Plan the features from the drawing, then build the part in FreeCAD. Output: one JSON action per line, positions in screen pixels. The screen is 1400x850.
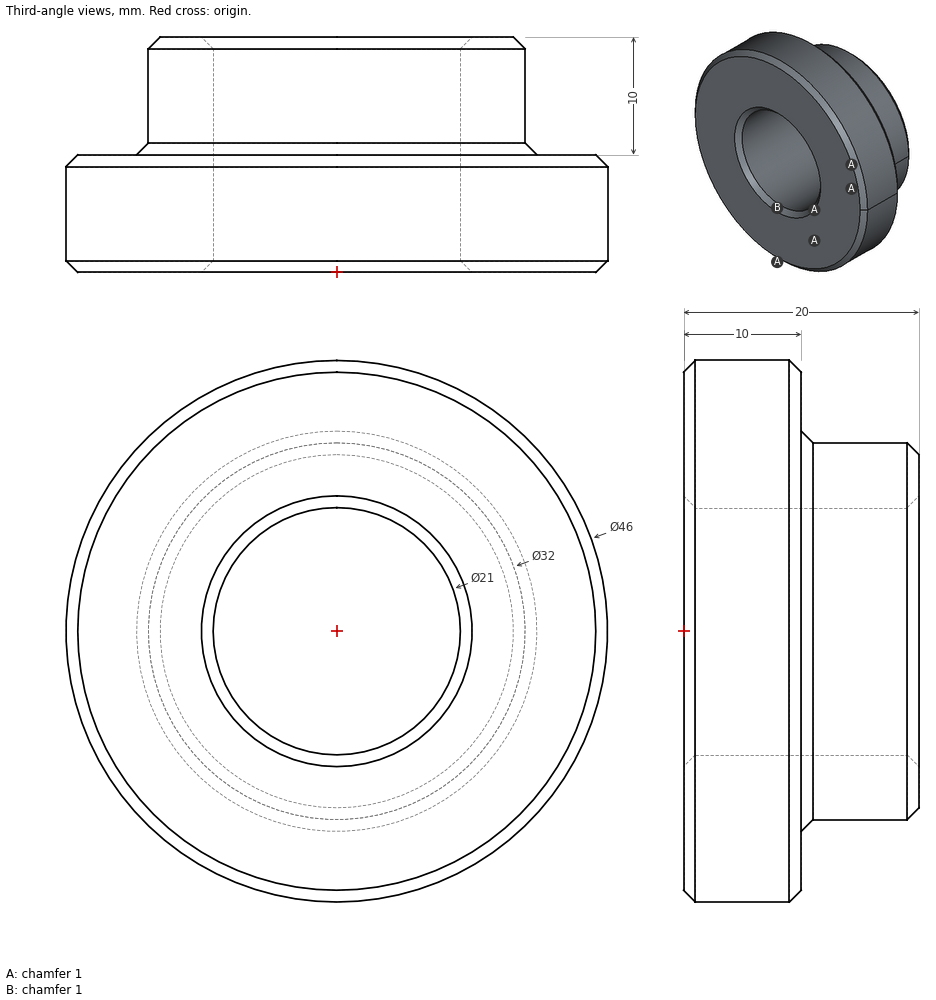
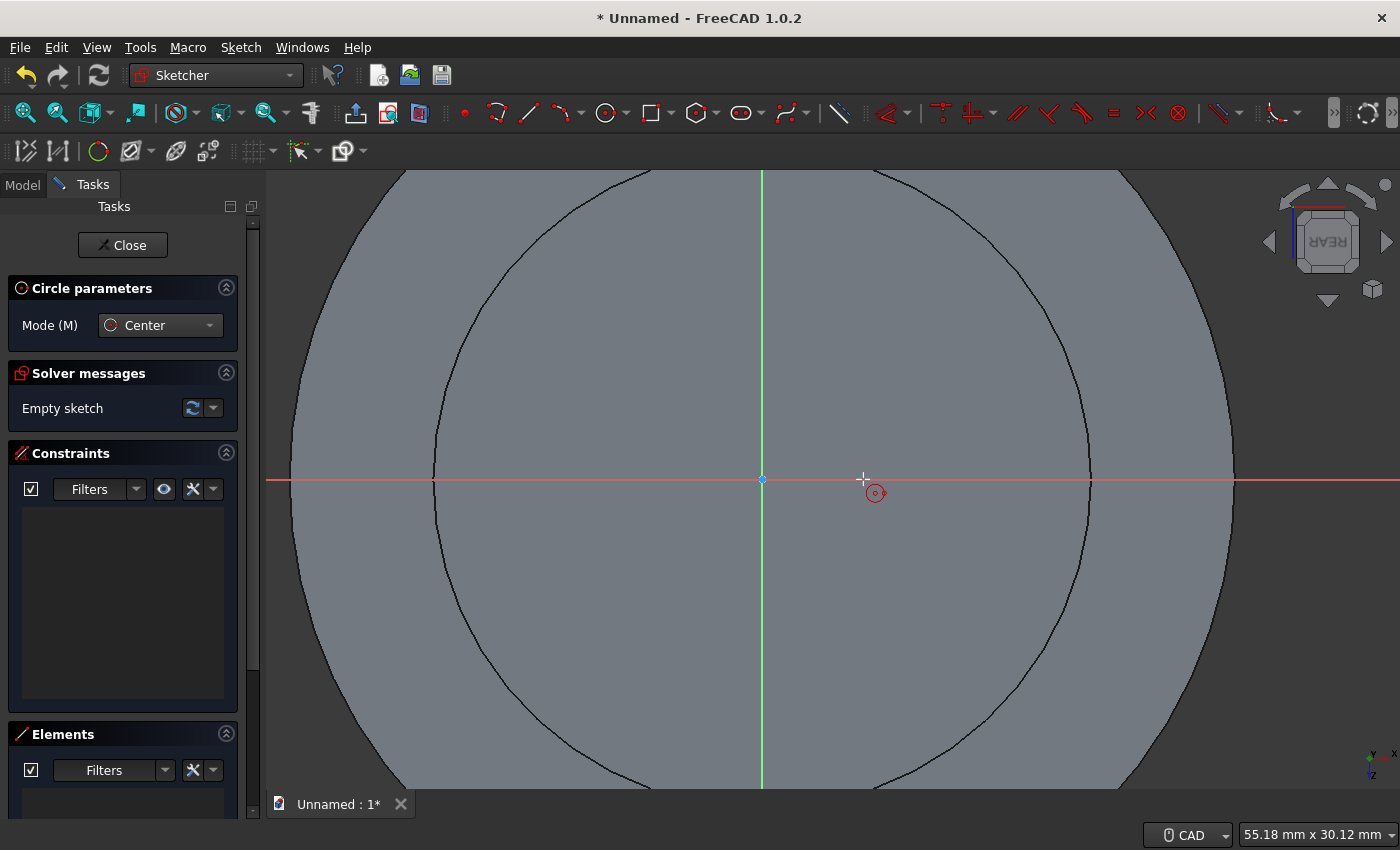
{"action": "left_click", "coordinate": [762, 479]}
{"action": "left_click", "coordinate": [915, 327]}
{"action": "key", "text": "Escape"}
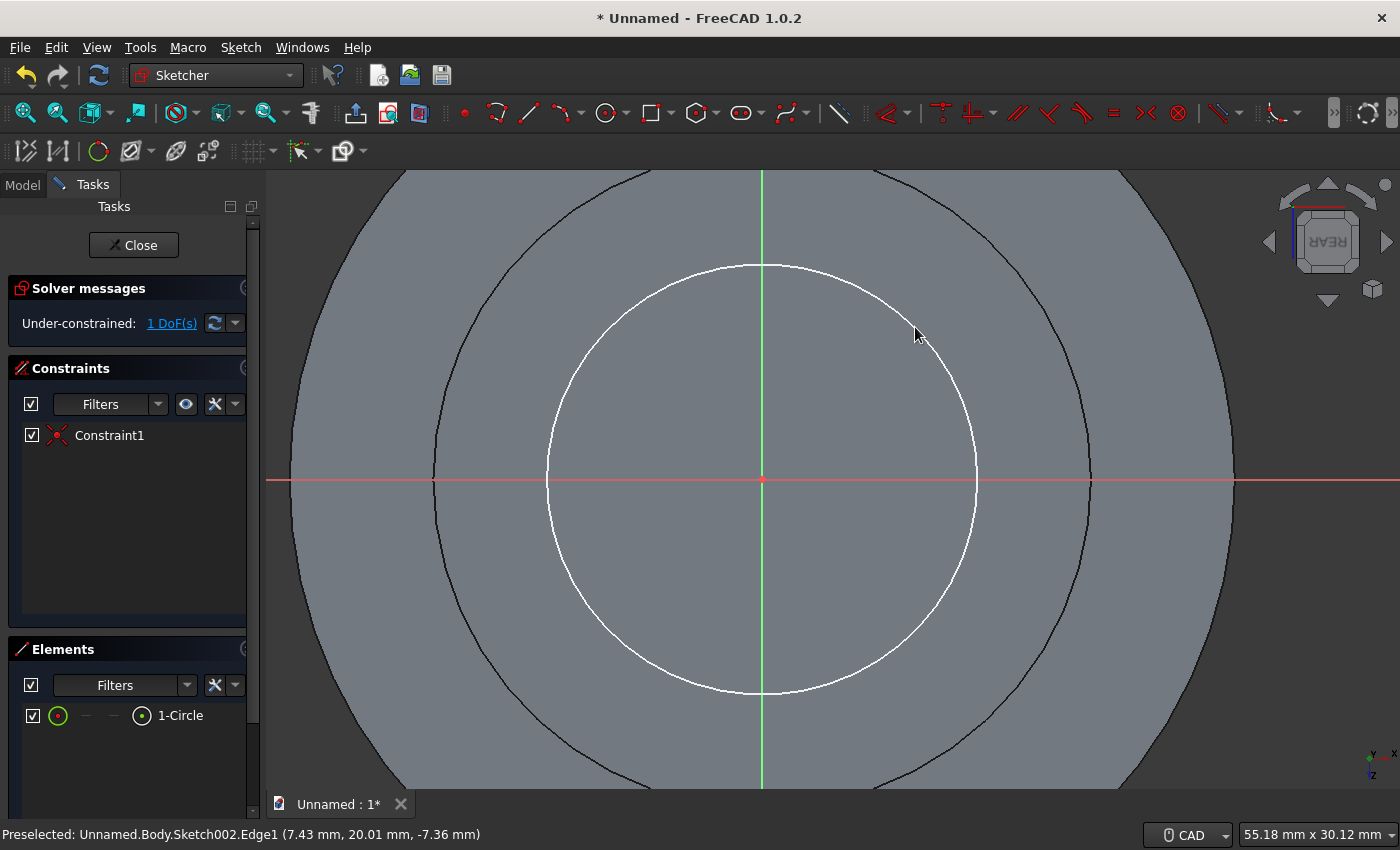
{"action": "key", "text": "d"}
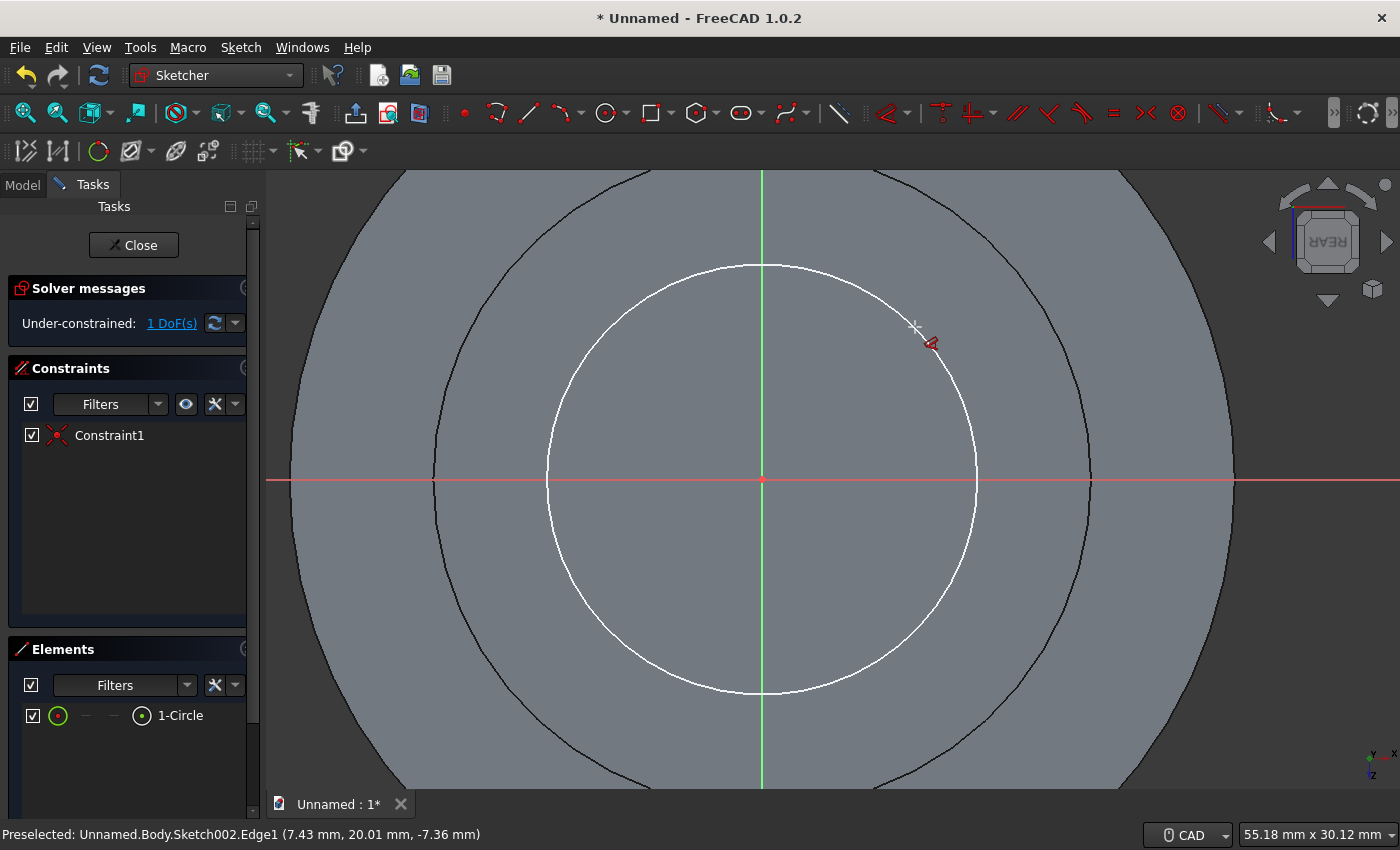
{"action": "left_click", "coordinate": [914, 327]}
{"action": "left_click", "coordinate": [937, 304]}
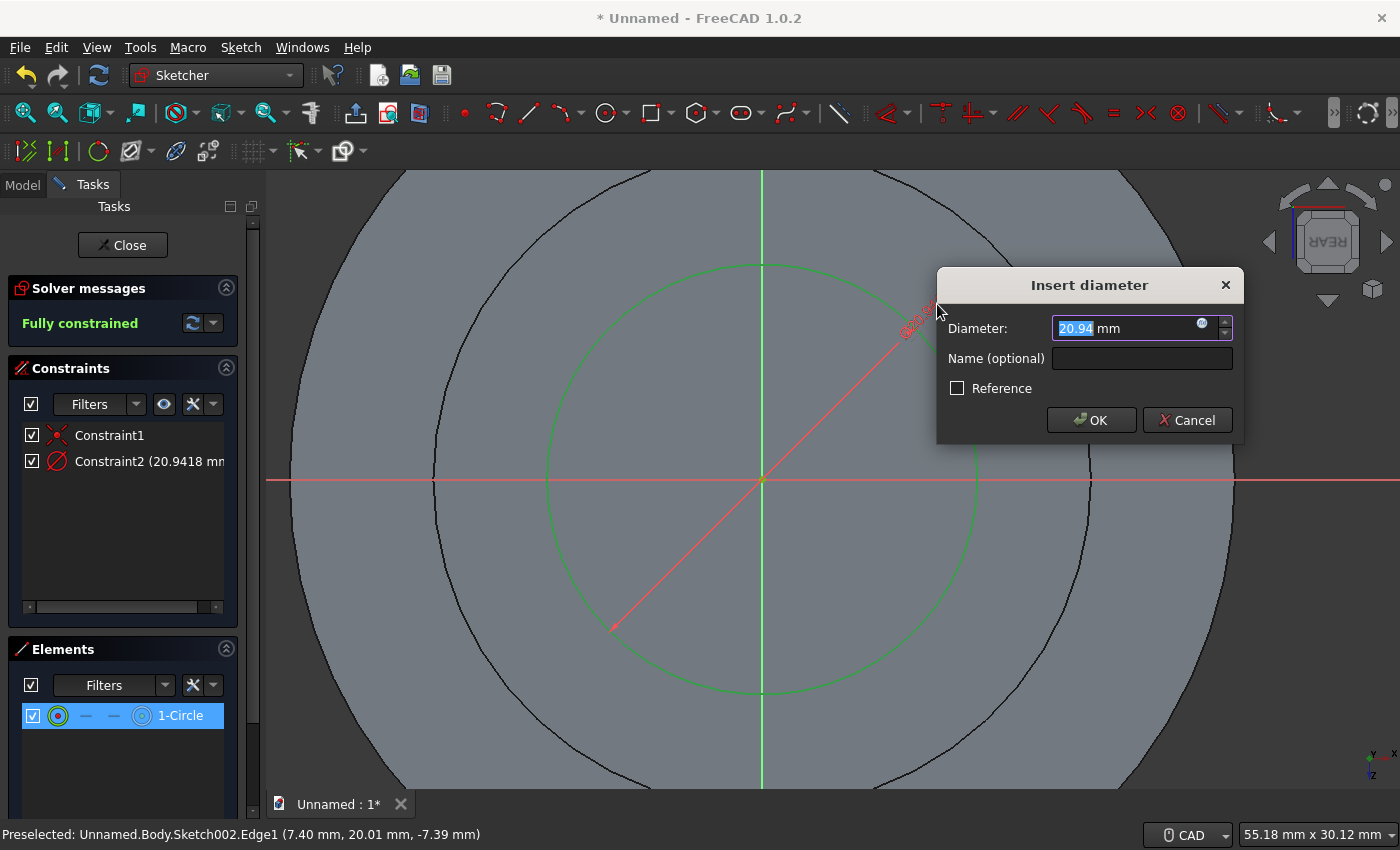
{"action": "type", "text": "21"}
{"action": "key", "text": "Return"}
{"action": "key", "text": "Escape"}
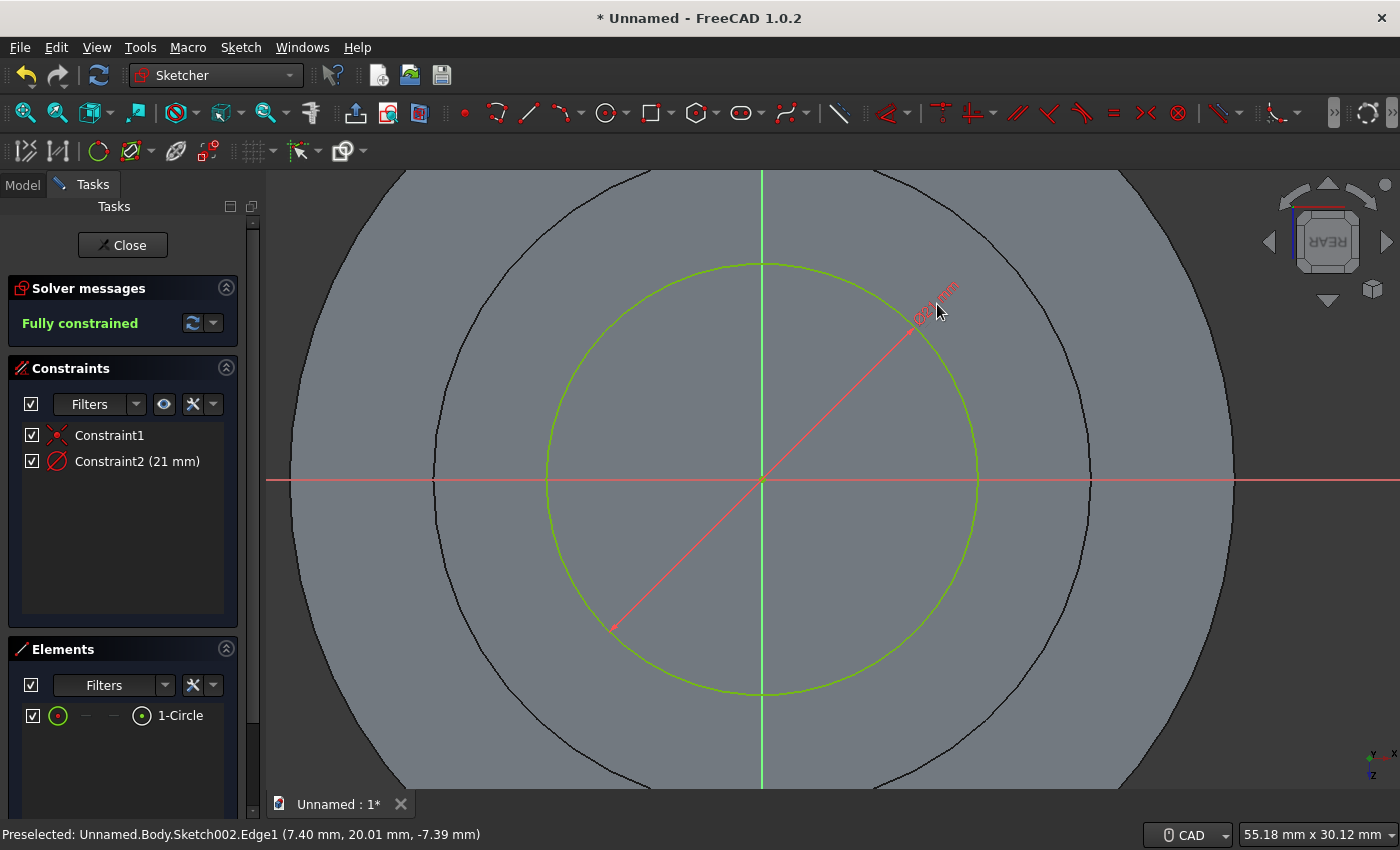
{"action": "left_click", "coordinate": [123, 245]}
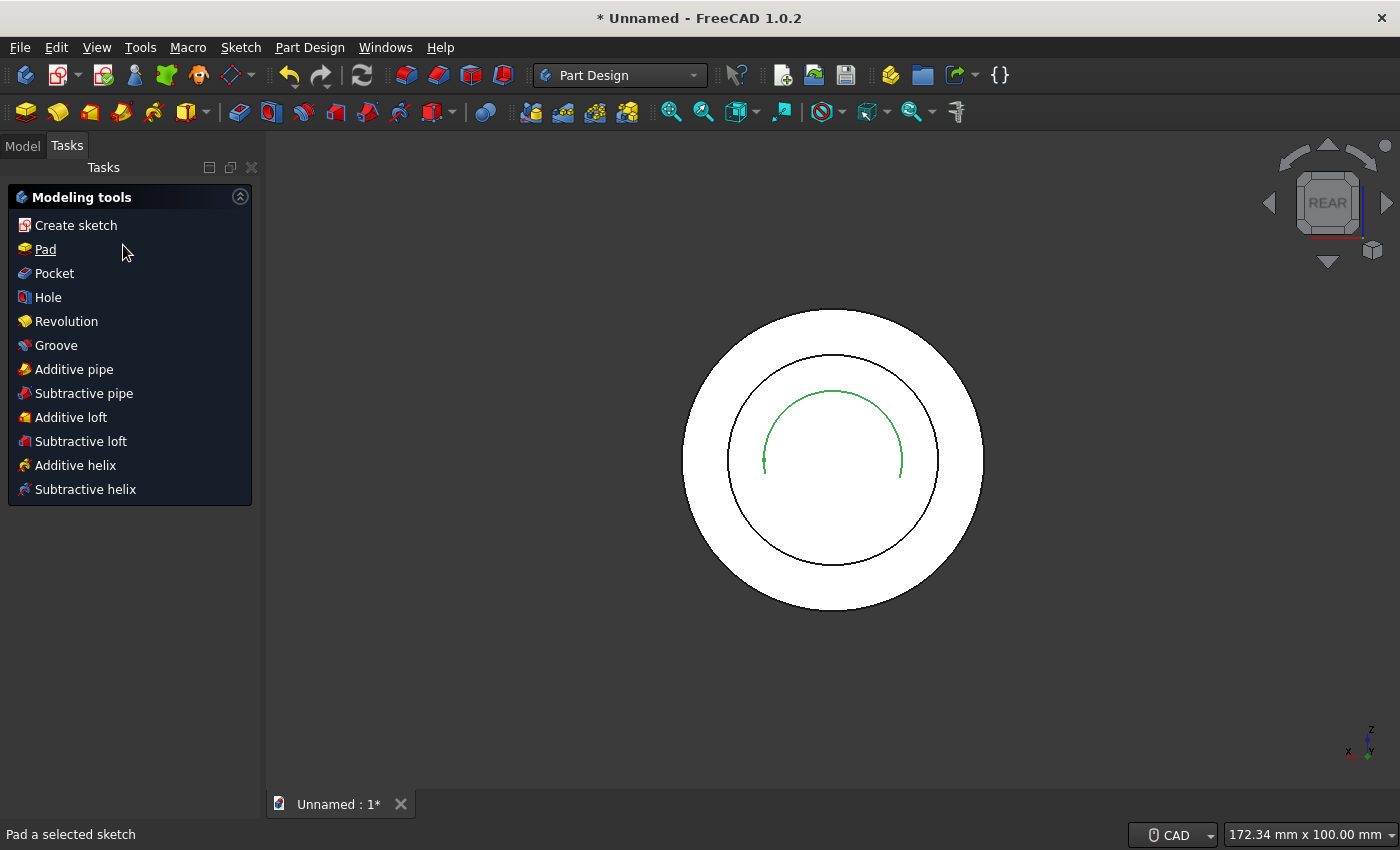
{"action": "left_click", "coordinate": [240, 112]}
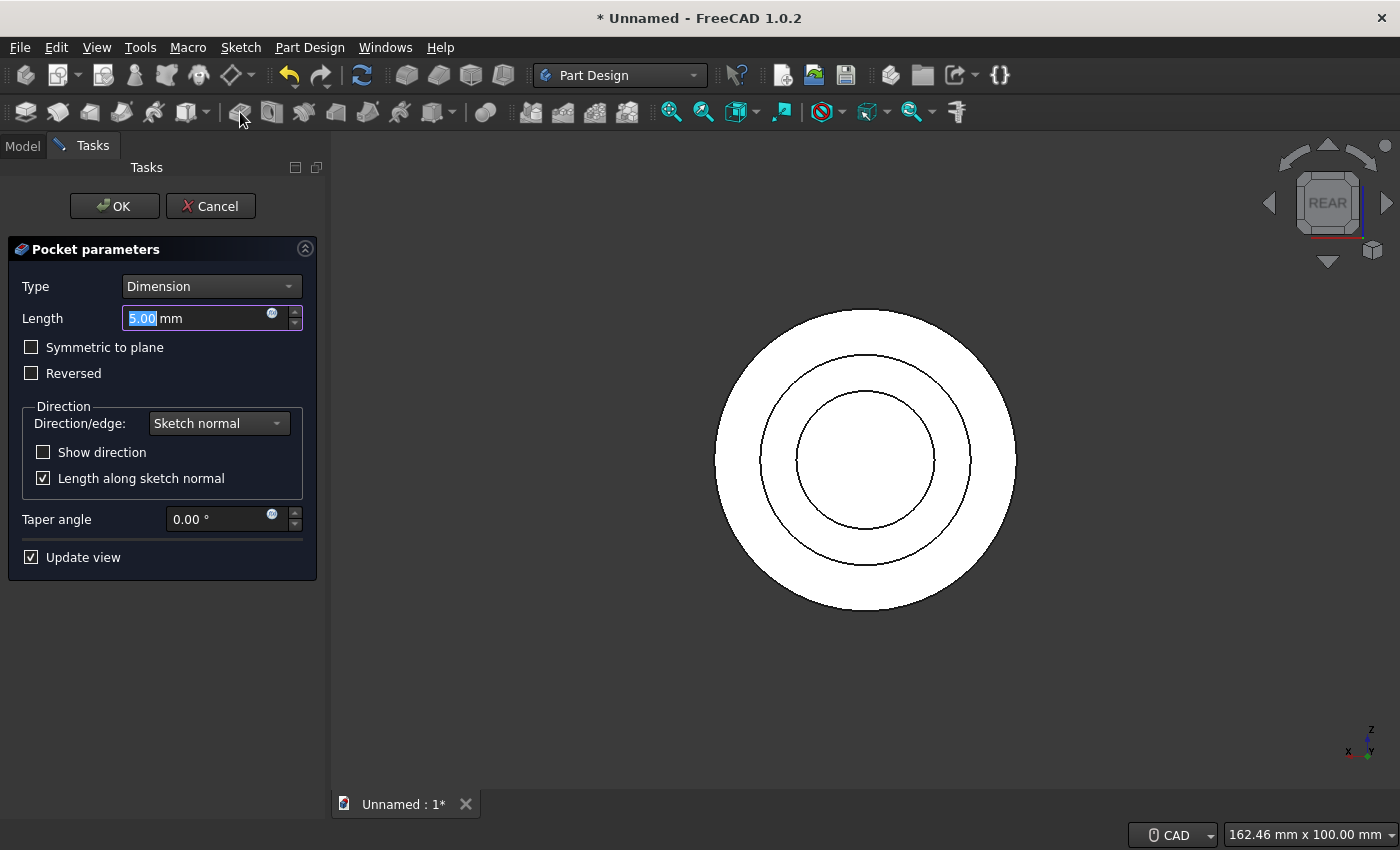
{"action": "type", "text": "20"}
{"action": "key", "text": "Tab"}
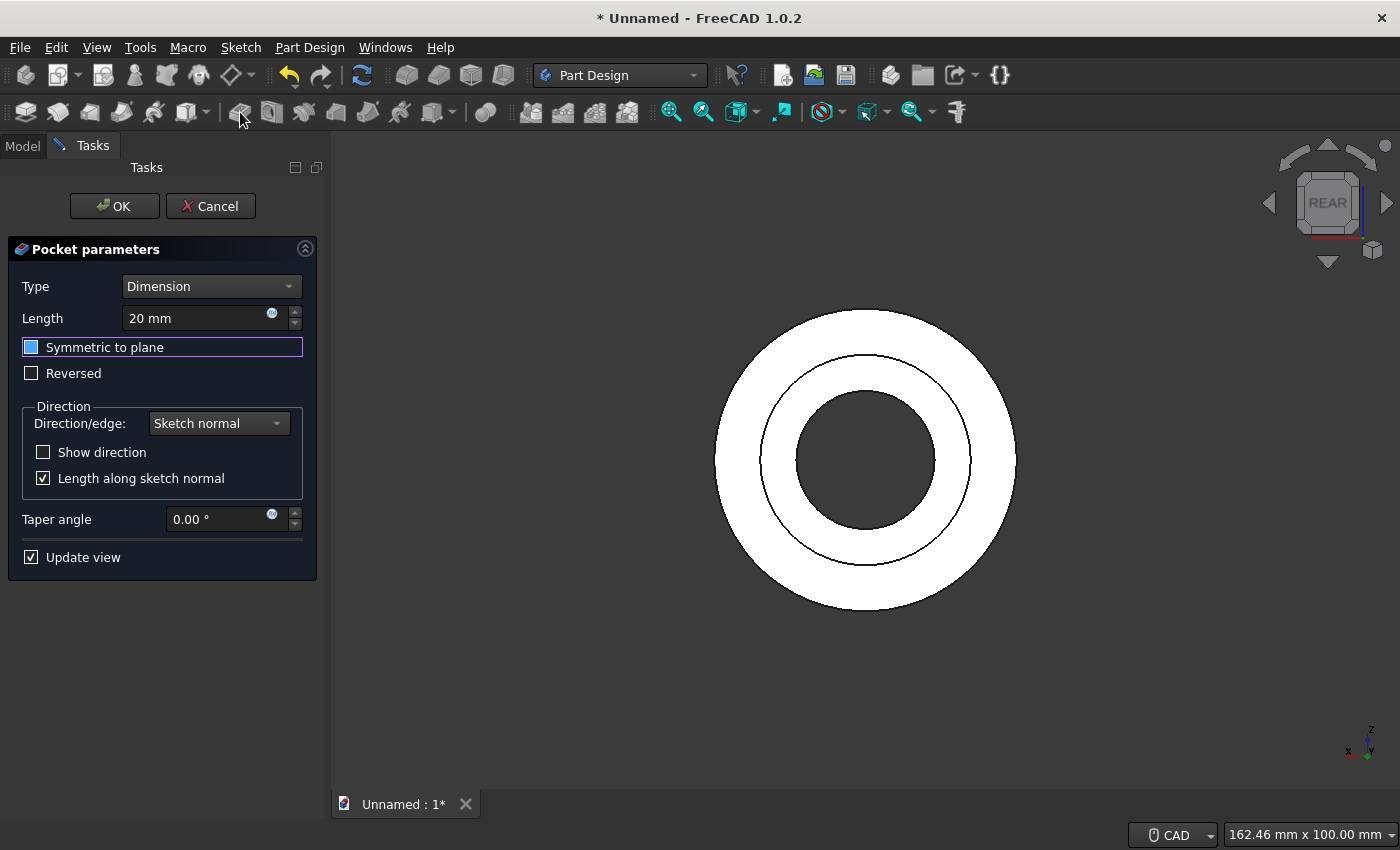
{"action": "left_click", "coordinate": [115, 206]}